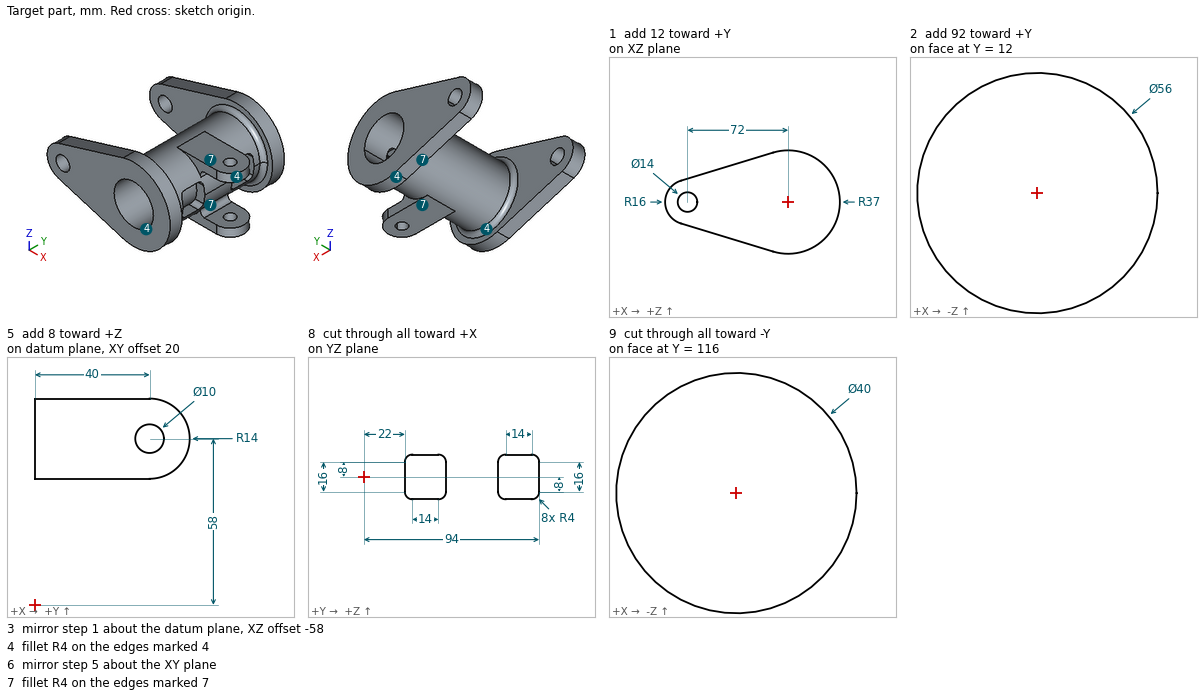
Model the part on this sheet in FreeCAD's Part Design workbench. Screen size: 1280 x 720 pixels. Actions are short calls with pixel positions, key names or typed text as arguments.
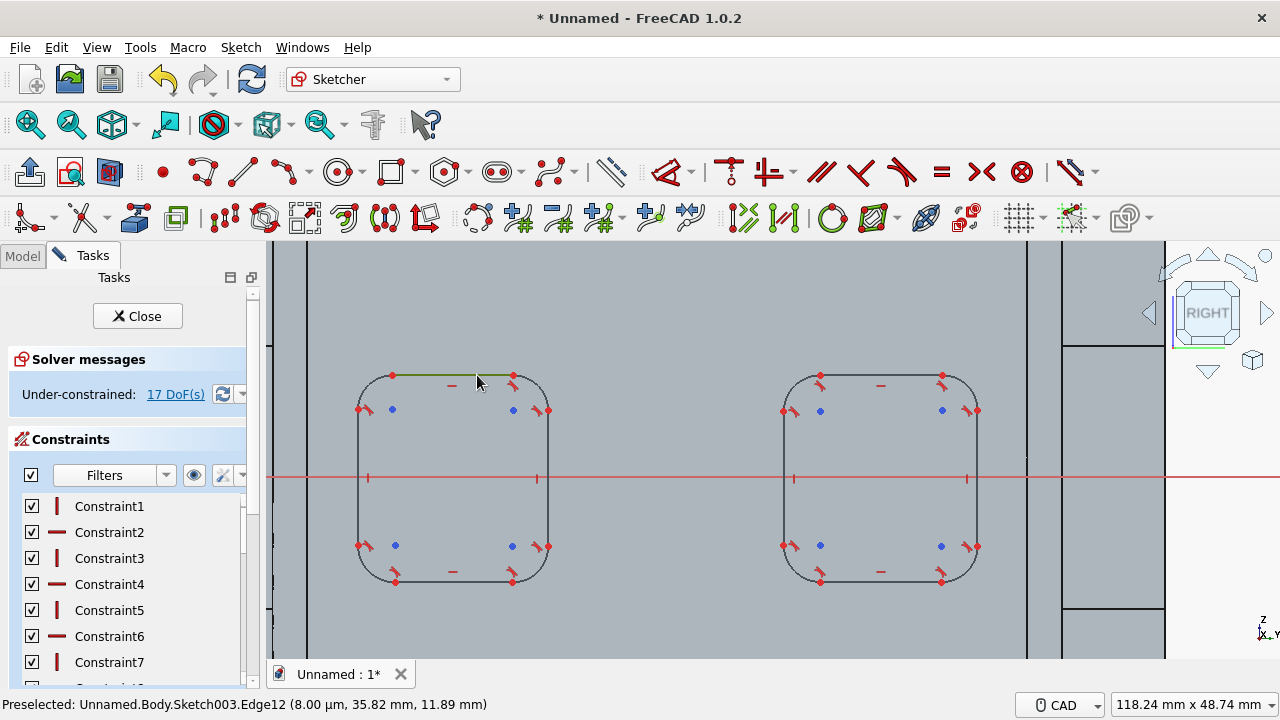
click(377, 379)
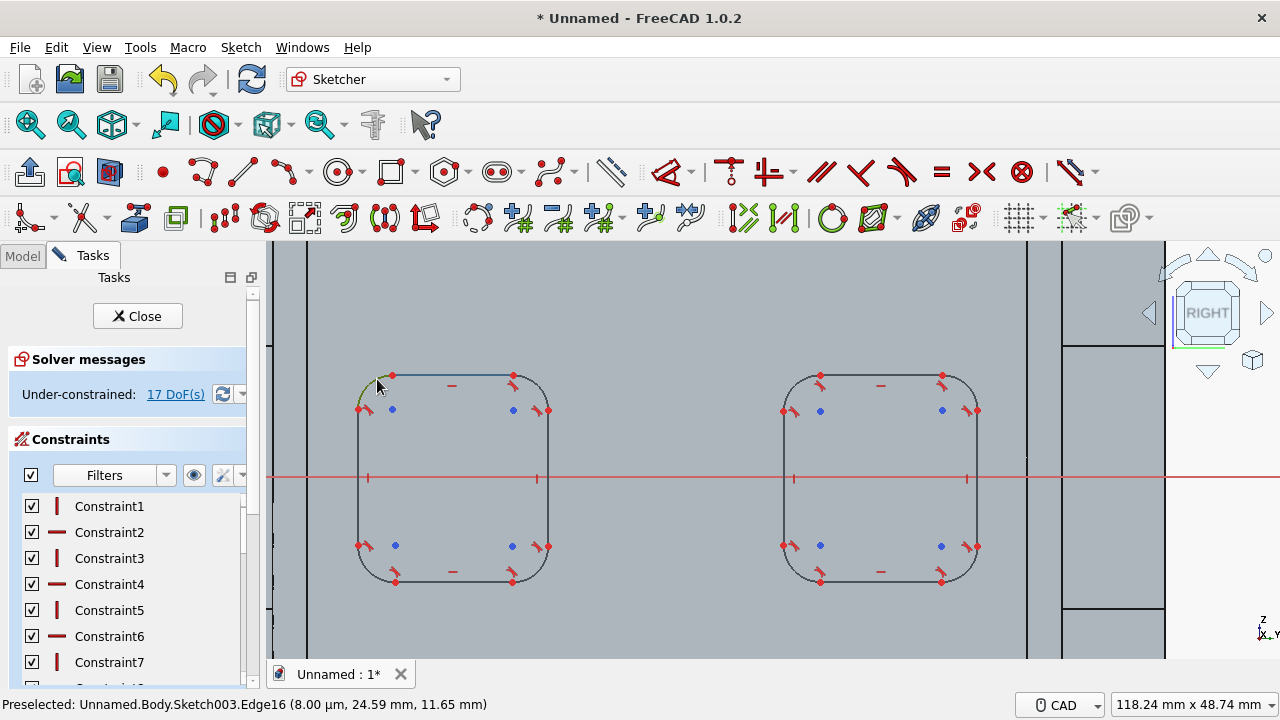
click(902, 172)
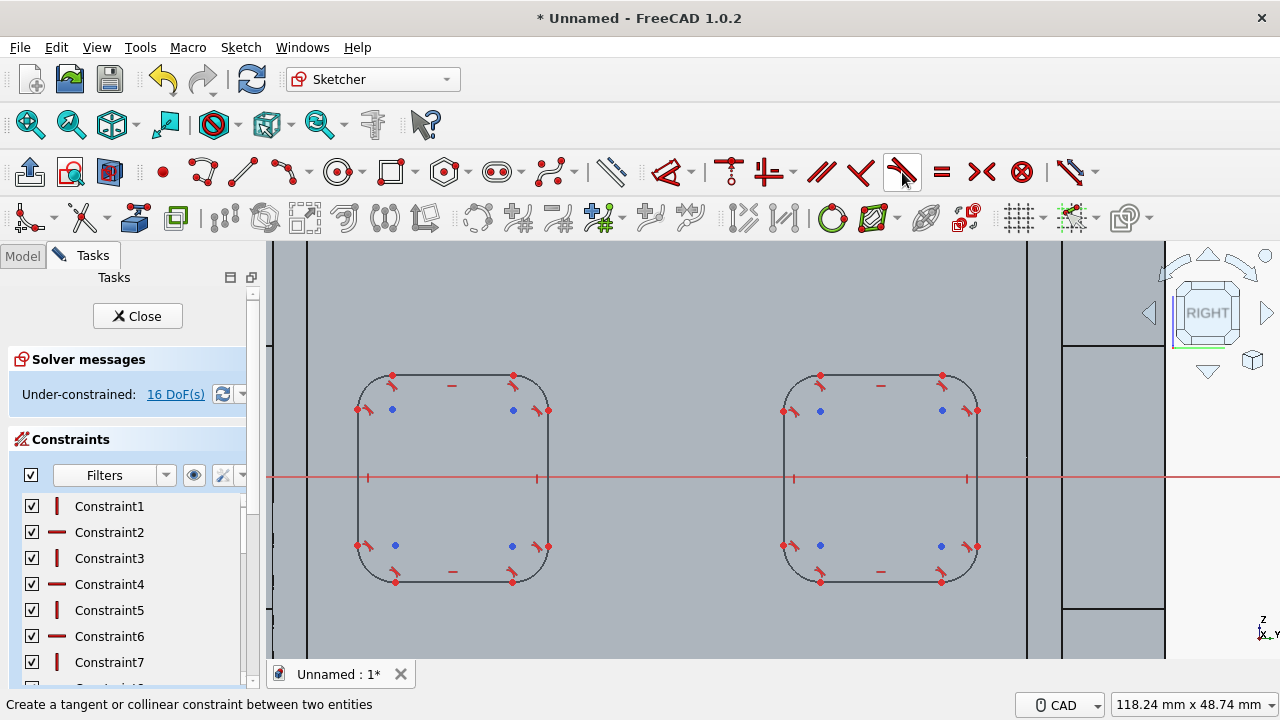
click(974, 394)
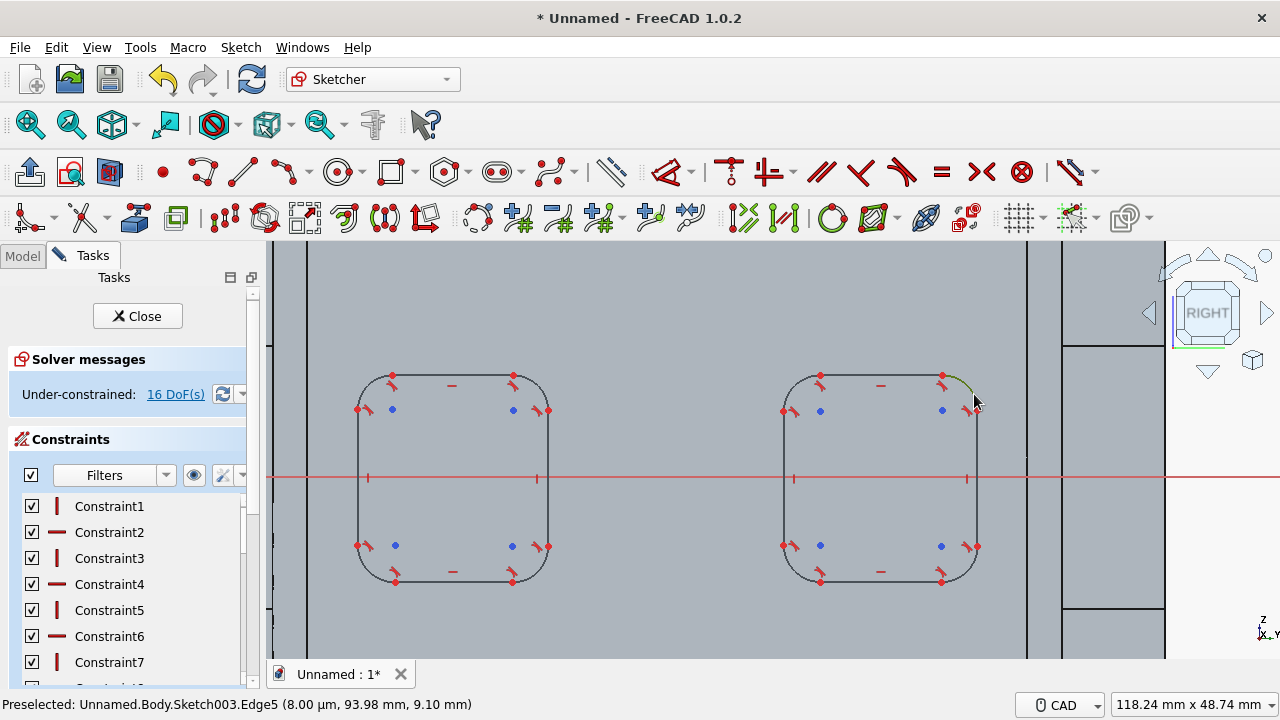
click(804, 379)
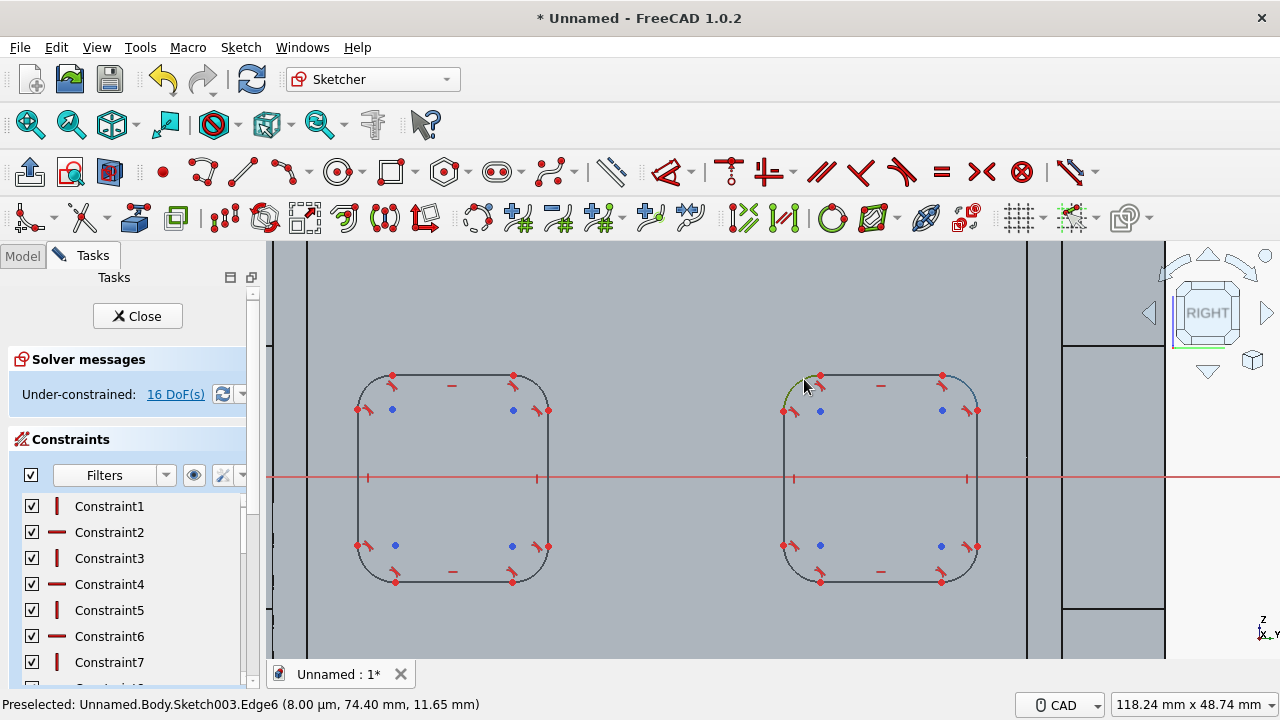
click(788, 562)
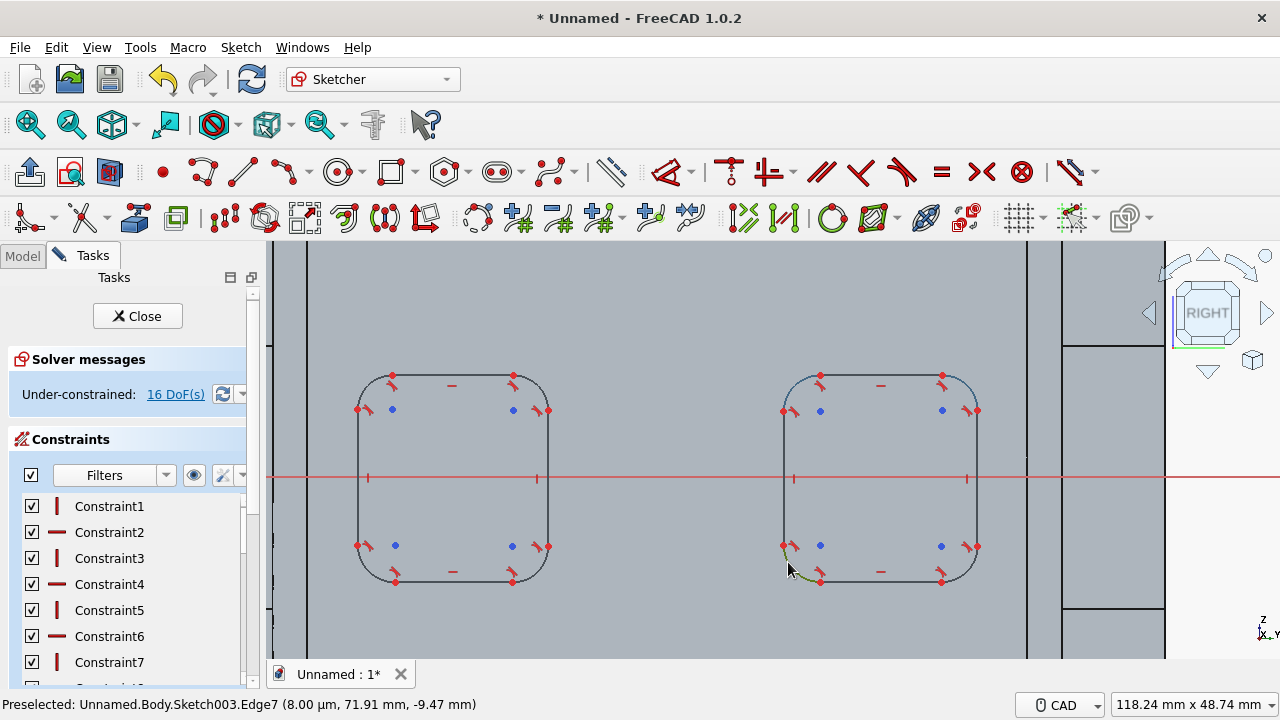
click(958, 578)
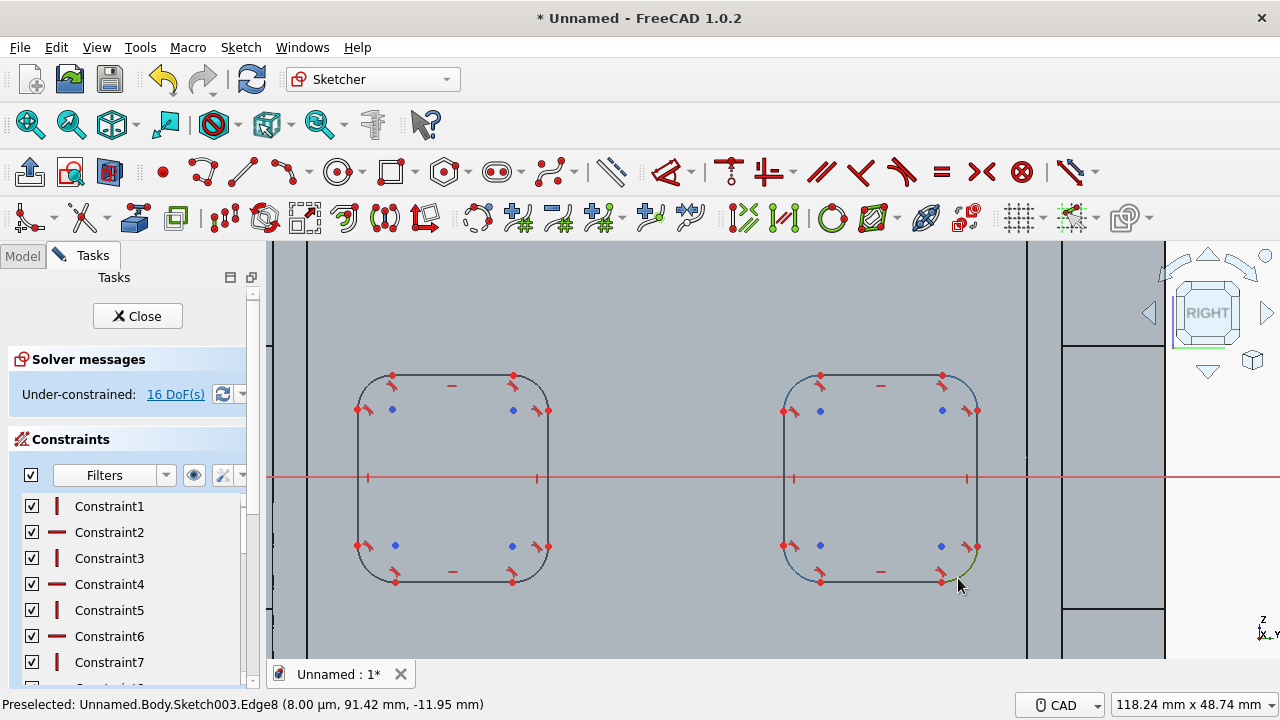
click(362, 562)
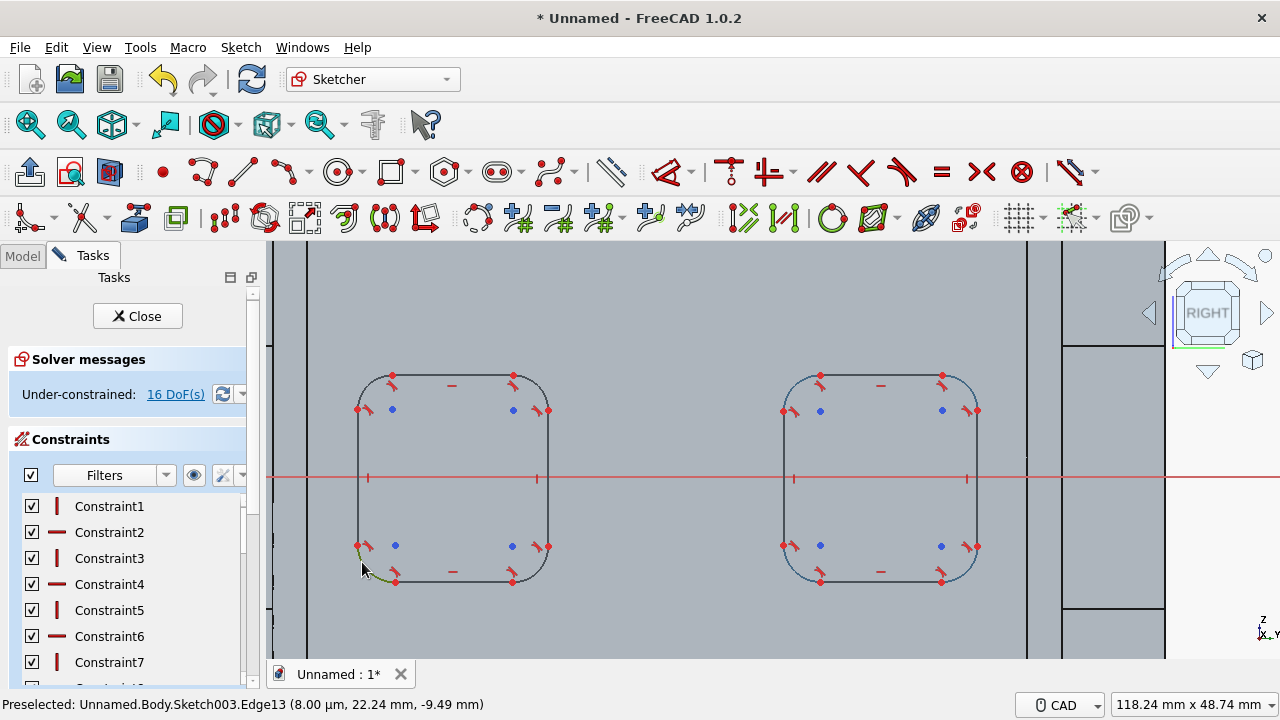
click(529, 578)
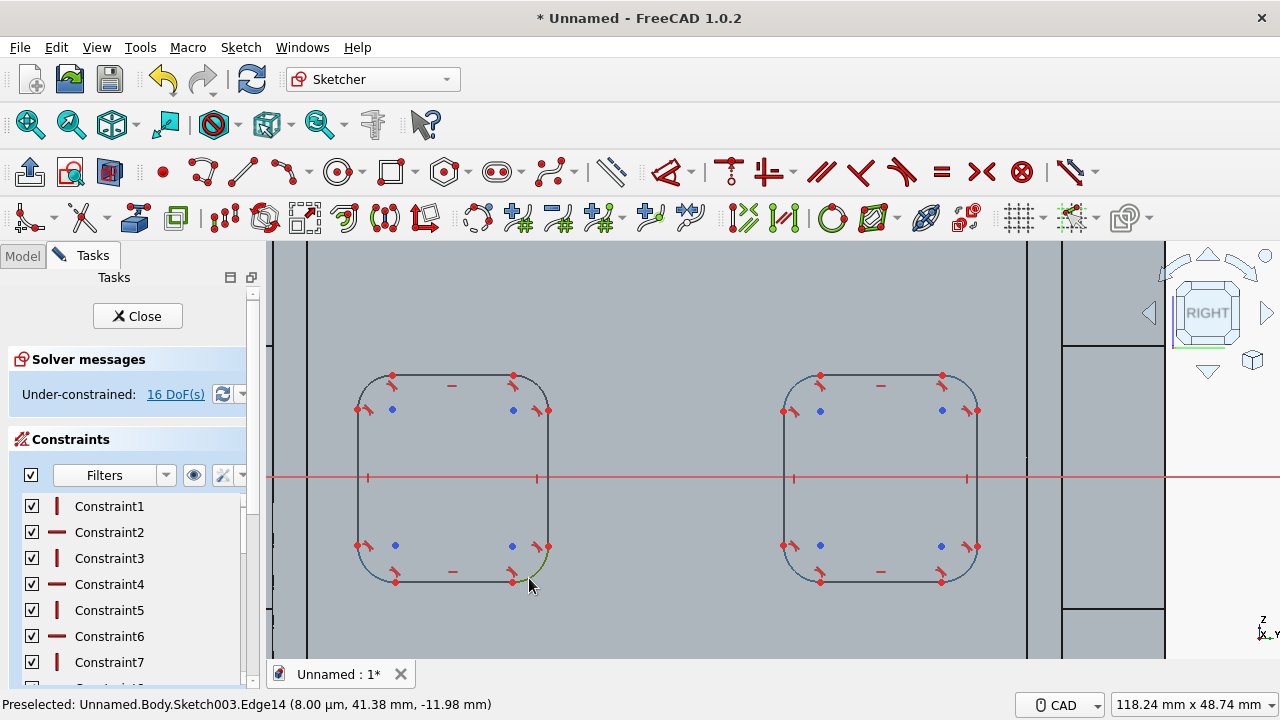
click(544, 394)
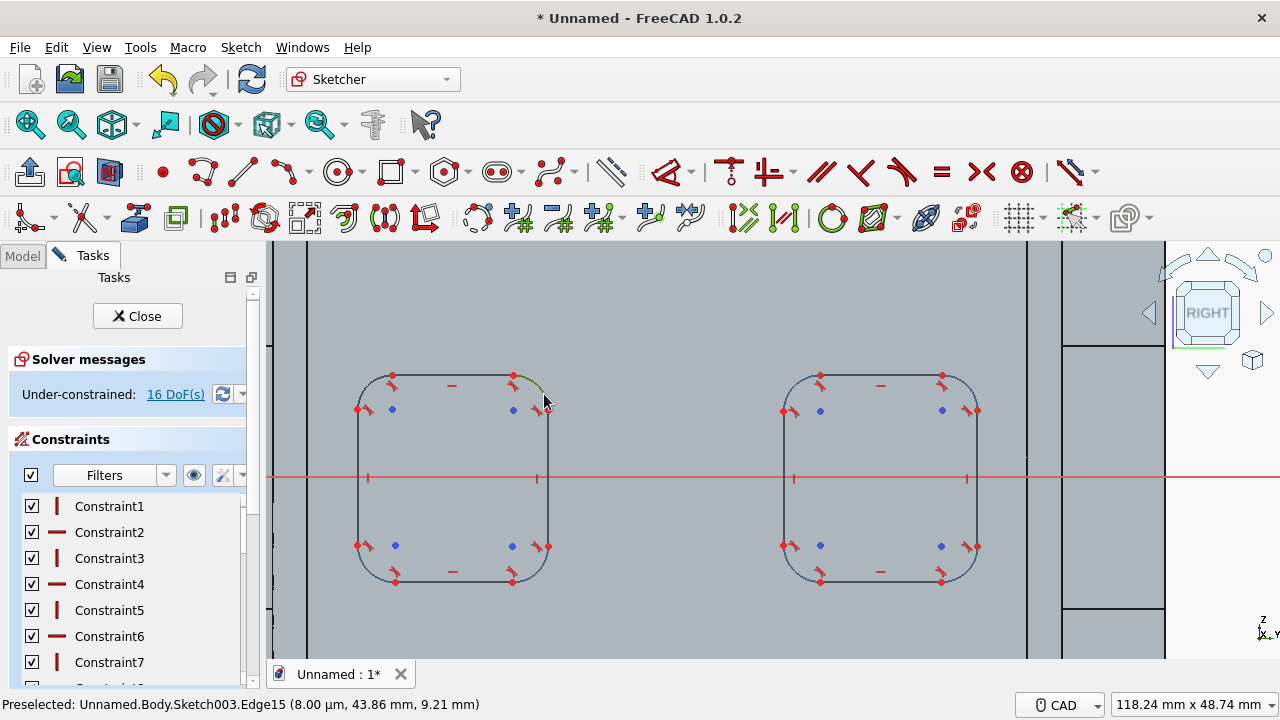
click(377, 379)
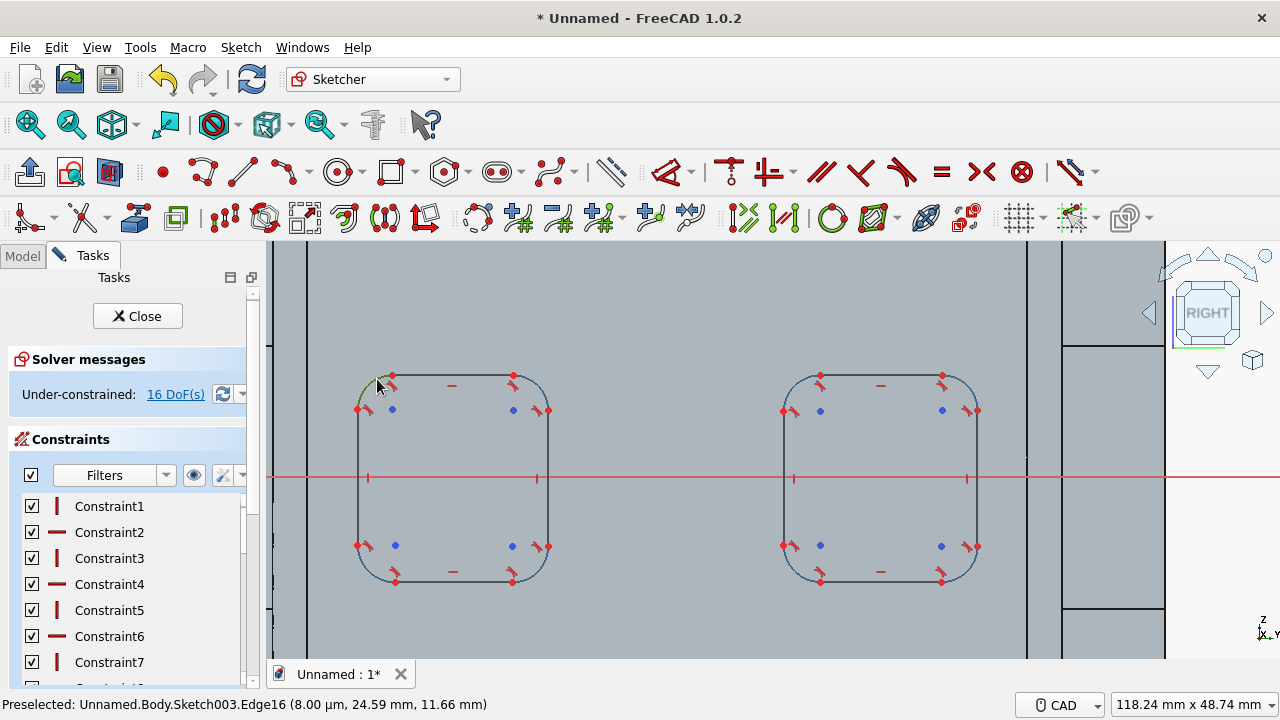
click(942, 172)